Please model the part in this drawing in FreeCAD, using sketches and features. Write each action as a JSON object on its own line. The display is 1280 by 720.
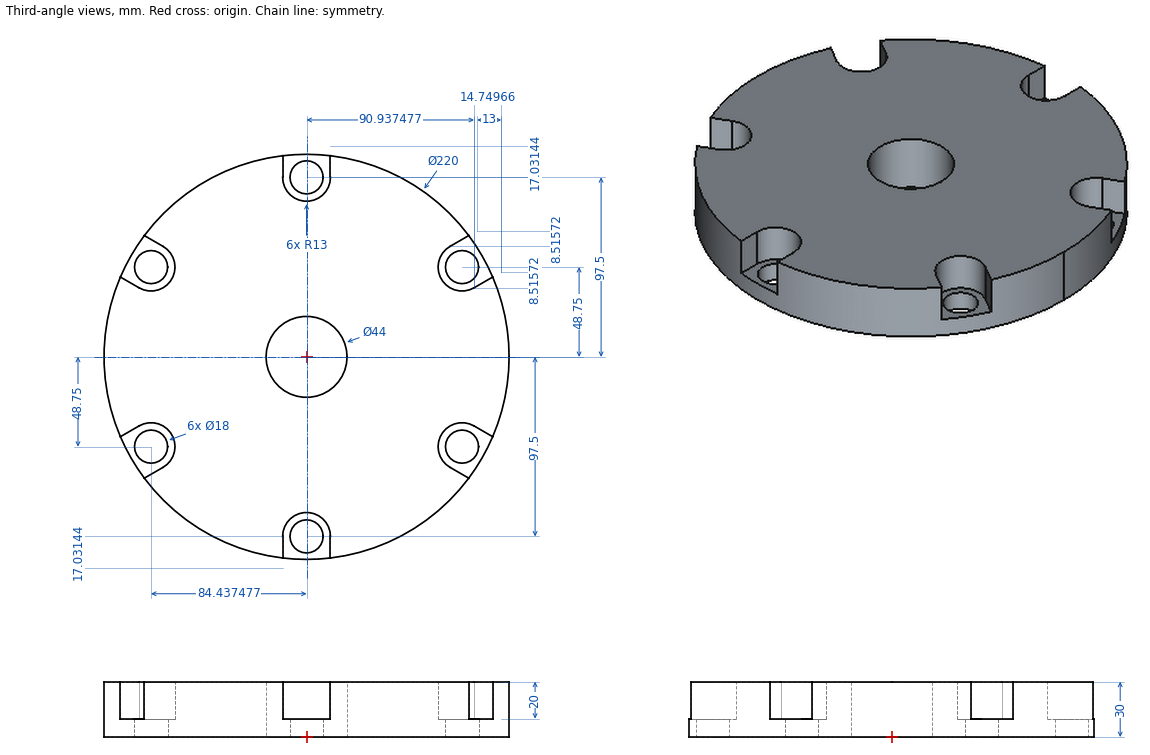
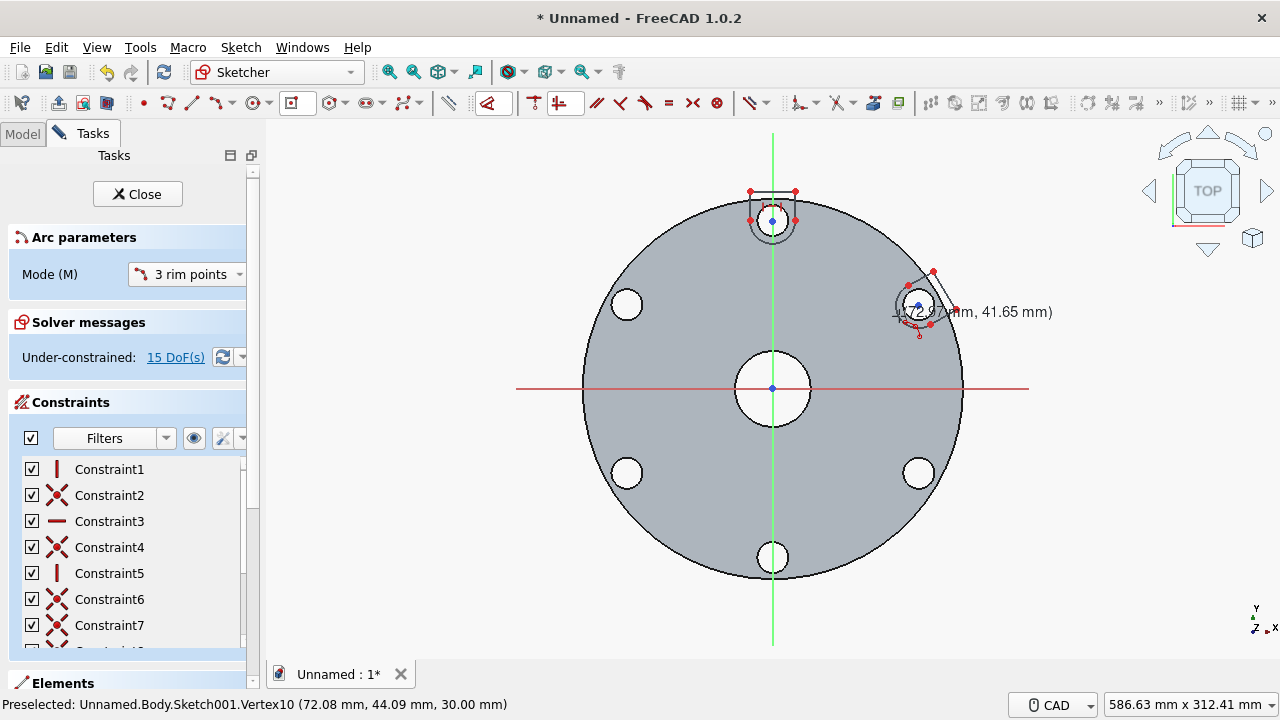
{"action": "left_click", "coordinate": [168, 104]}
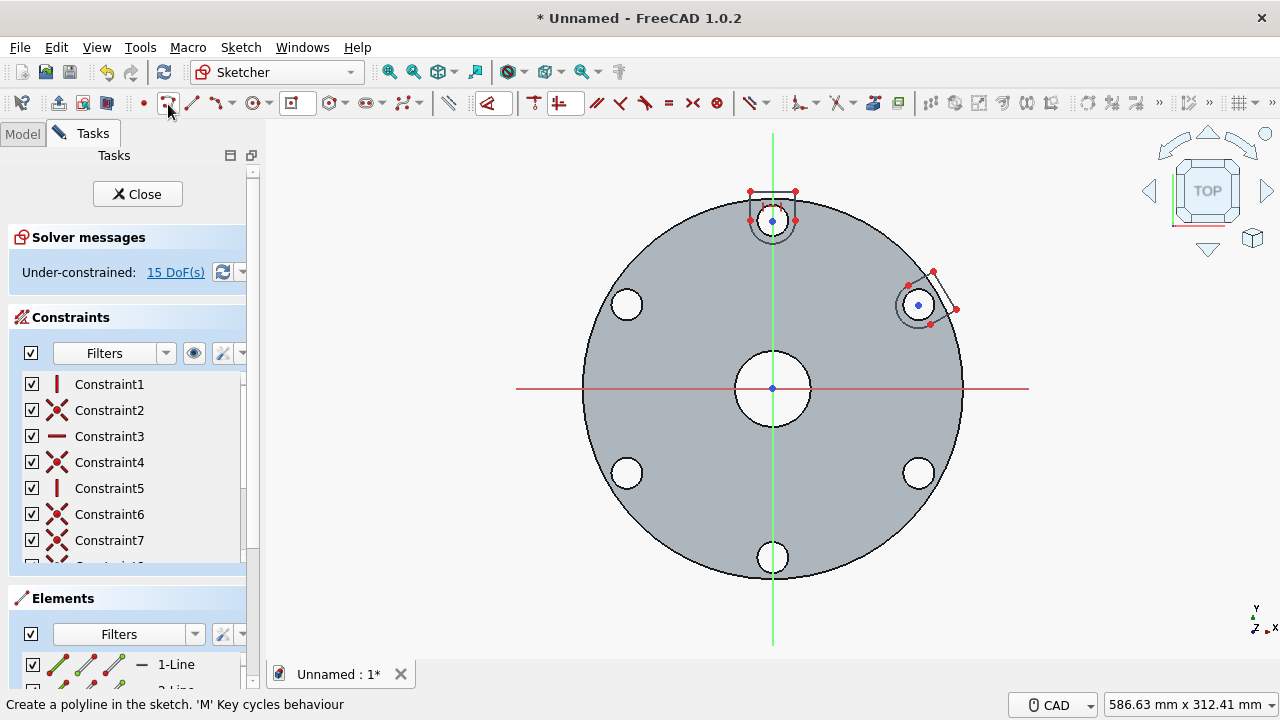
{"action": "left_click", "coordinate": [908, 493]}
{"action": "left_click", "coordinate": [933, 507]}
{"action": "left_click", "coordinate": [956, 469]}
{"action": "left_click", "coordinate": [930, 454]}
{"action": "right_click", "coordinate": [930, 454]}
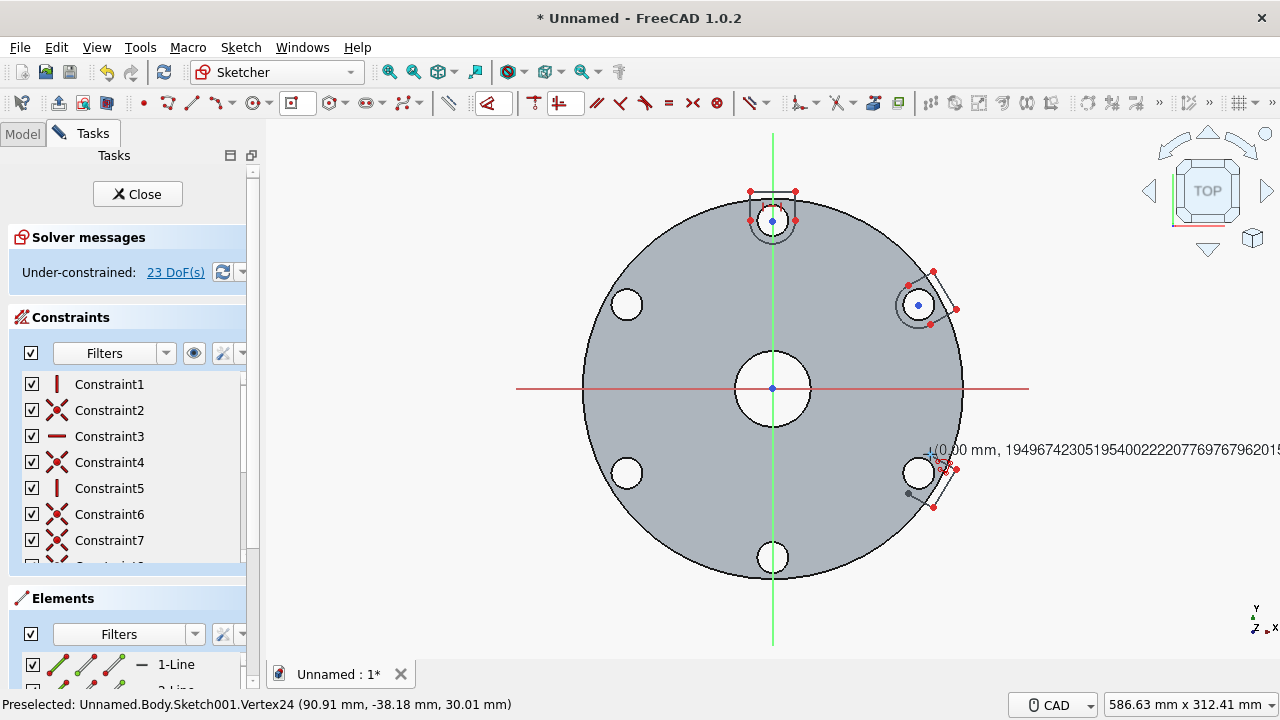
{"action": "left_click", "coordinate": [216, 104]}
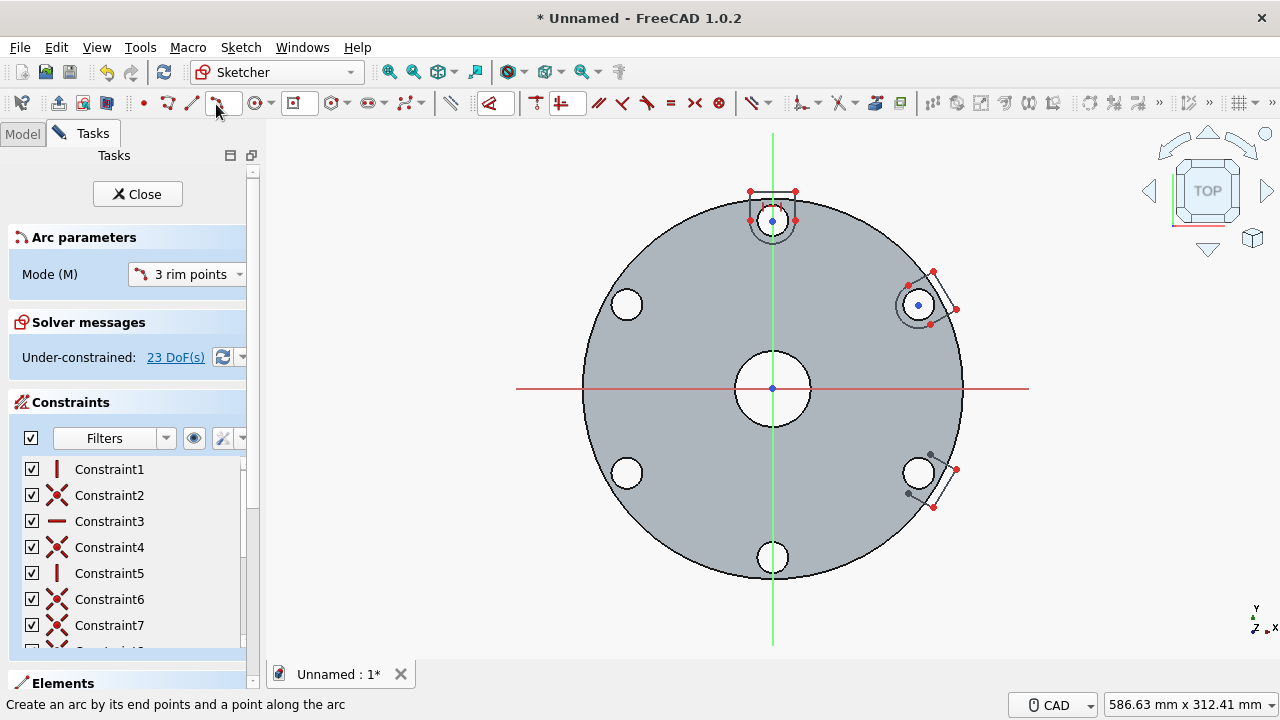
{"action": "left_click", "coordinate": [930, 455]}
{"action": "left_click", "coordinate": [908, 494]}
{"action": "left_click", "coordinate": [899, 462]}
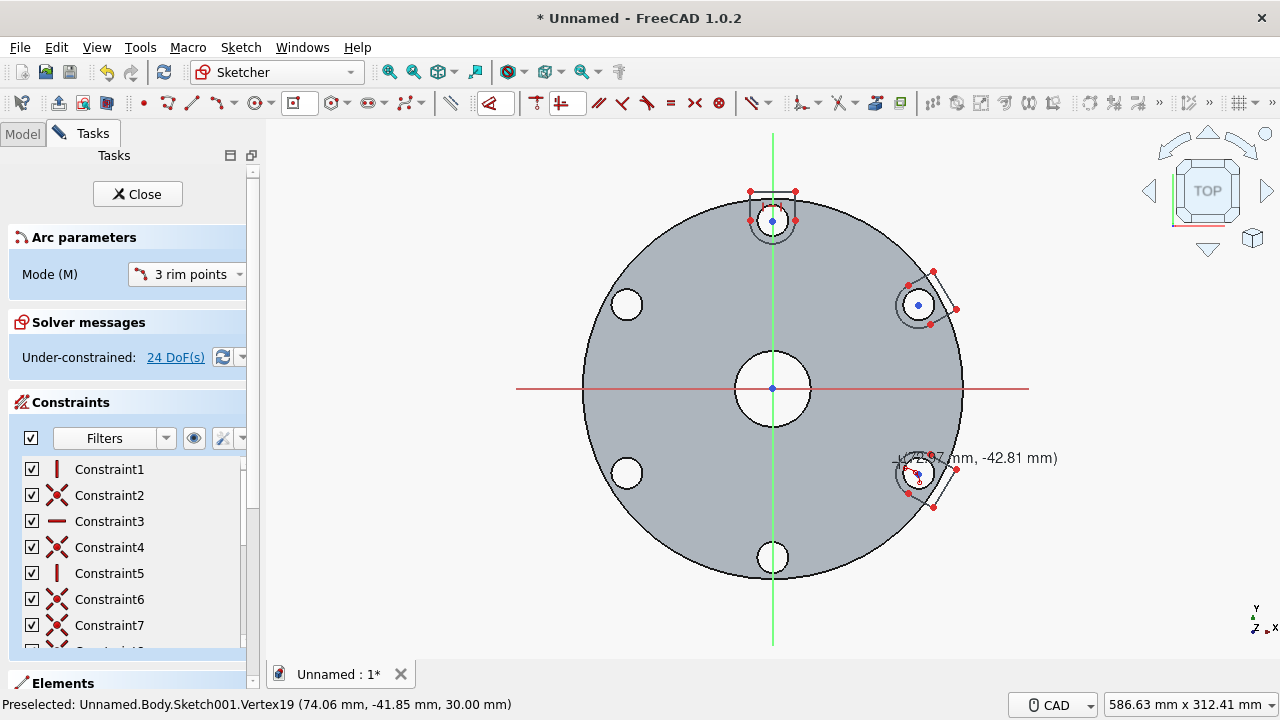
{"action": "key", "text": "g m"}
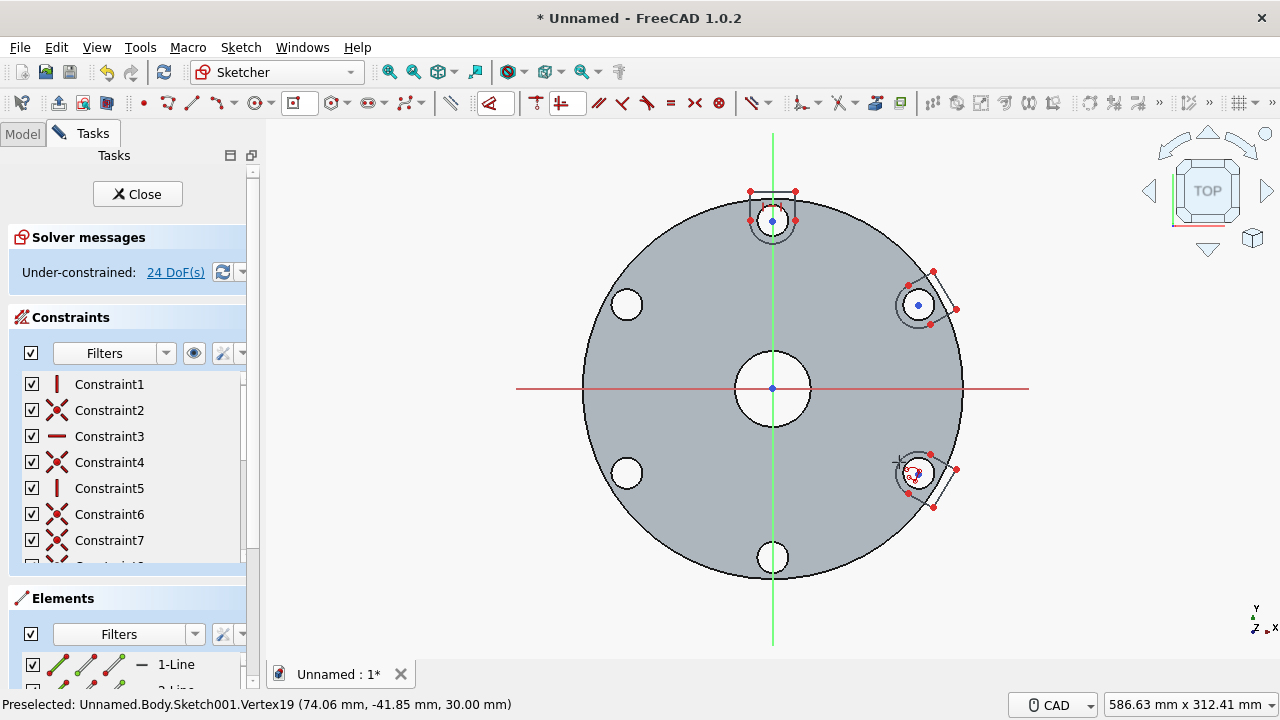
{"action": "left_click", "coordinate": [750, 558]}
{"action": "left_click", "coordinate": [750, 587]}
{"action": "left_click", "coordinate": [795, 587]}
{"action": "left_click", "coordinate": [795, 558]}
{"action": "right_click", "coordinate": [795, 558]}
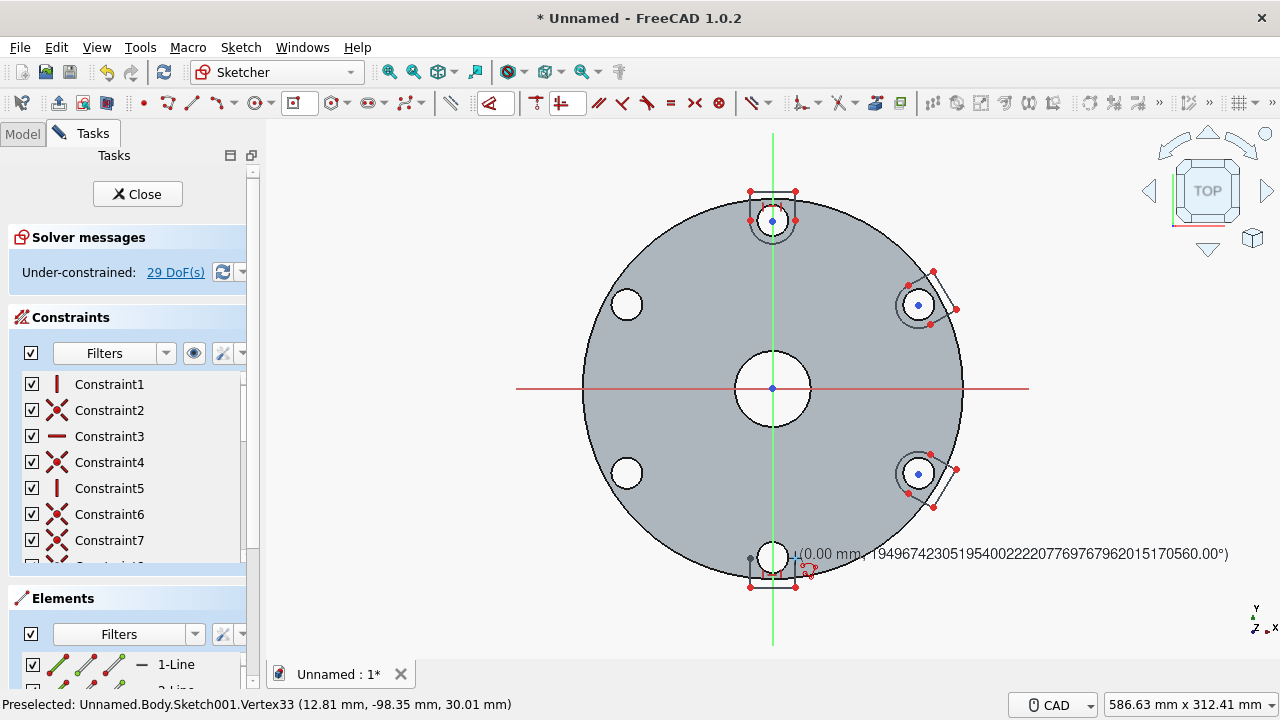
{"action": "left_click", "coordinate": [218, 104]}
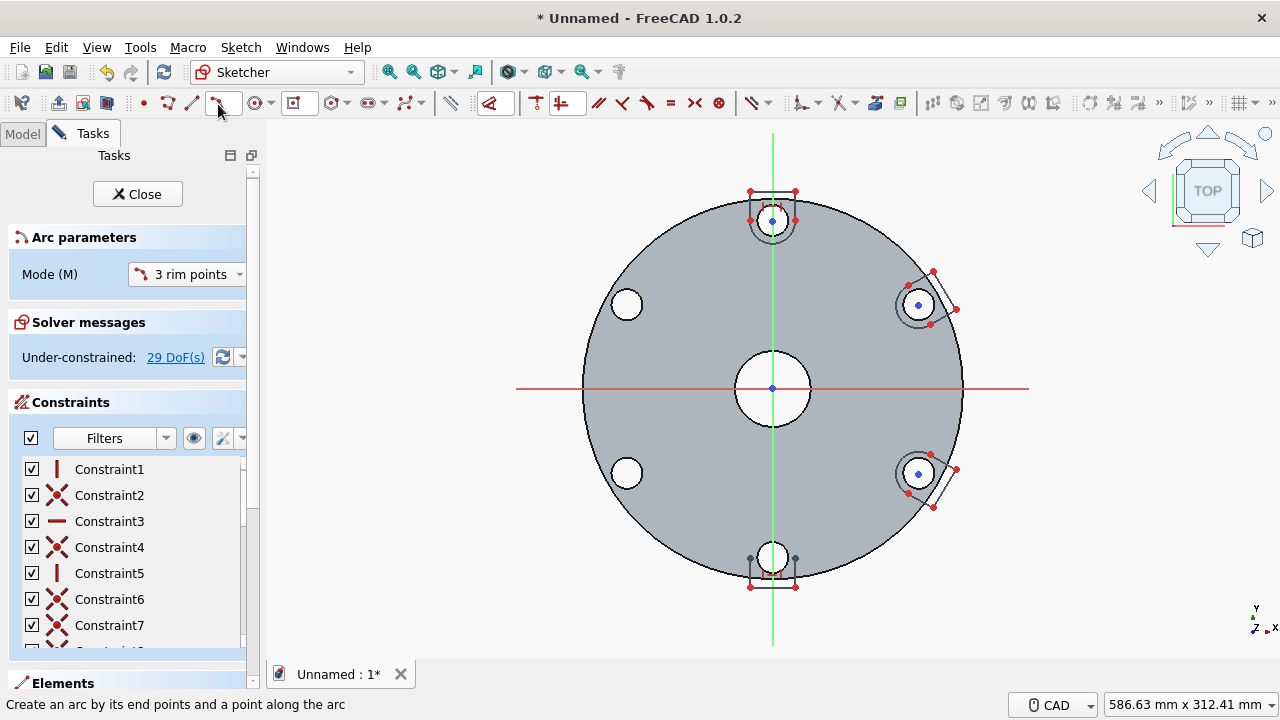
{"action": "left_click", "coordinate": [795, 559]}
{"action": "left_click", "coordinate": [750, 559]}
{"action": "left_click", "coordinate": [786, 539]}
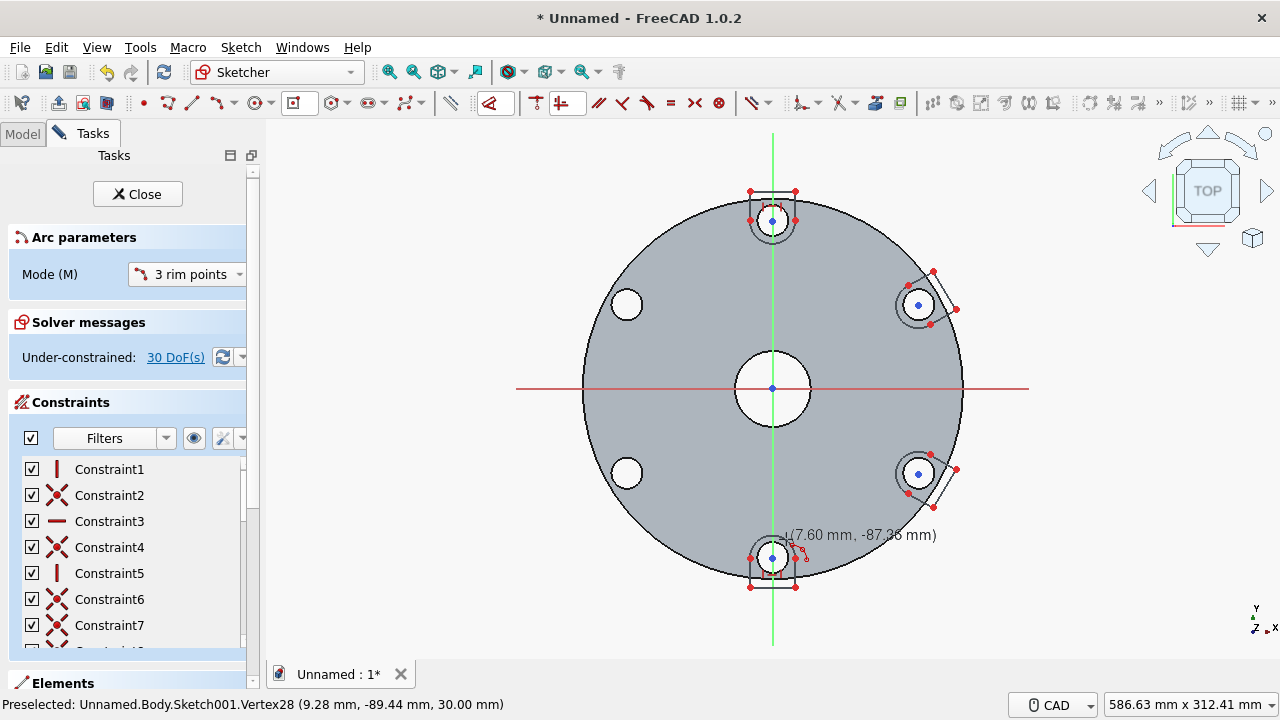
{"action": "key", "text": "g m"}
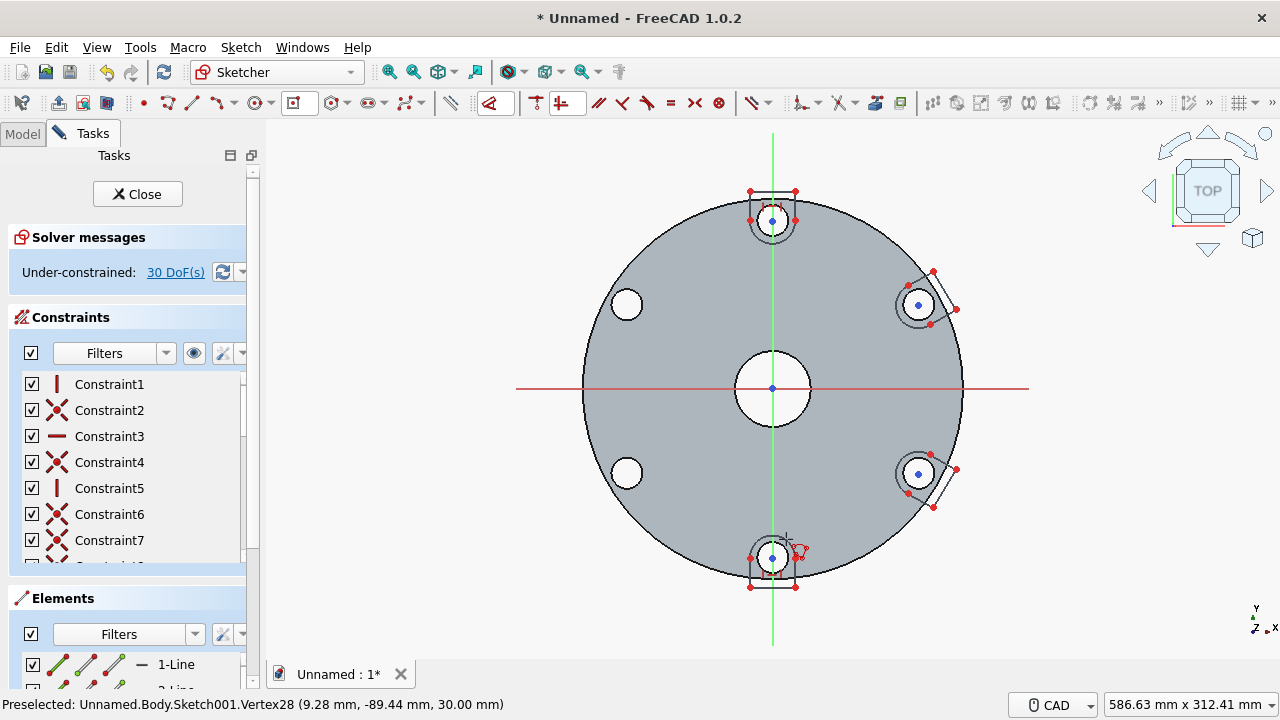
{"action": "left_click", "coordinate": [616, 454]}
{"action": "left_click", "coordinate": [590, 469]}
{"action": "left_click", "coordinate": [613, 507]}
{"action": "left_click", "coordinate": [638, 493]}
{"action": "right_click", "coordinate": [638, 493]}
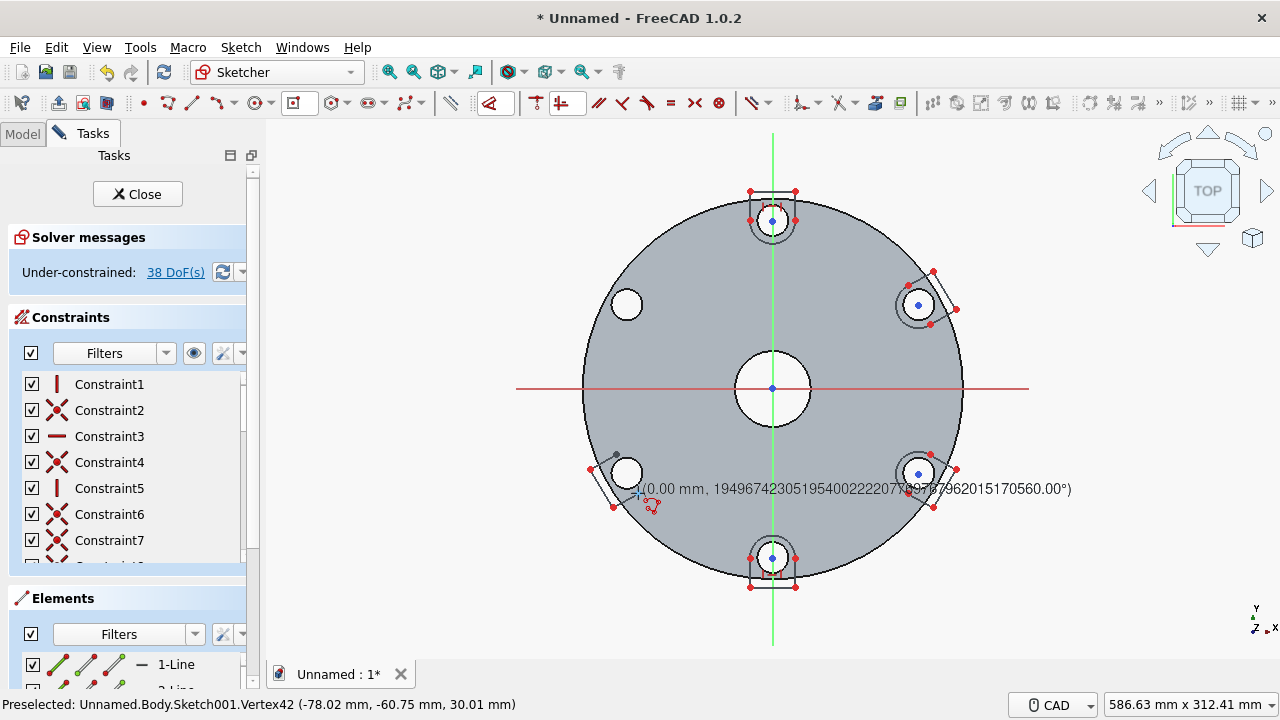
{"action": "key", "text": "g 3 a"}